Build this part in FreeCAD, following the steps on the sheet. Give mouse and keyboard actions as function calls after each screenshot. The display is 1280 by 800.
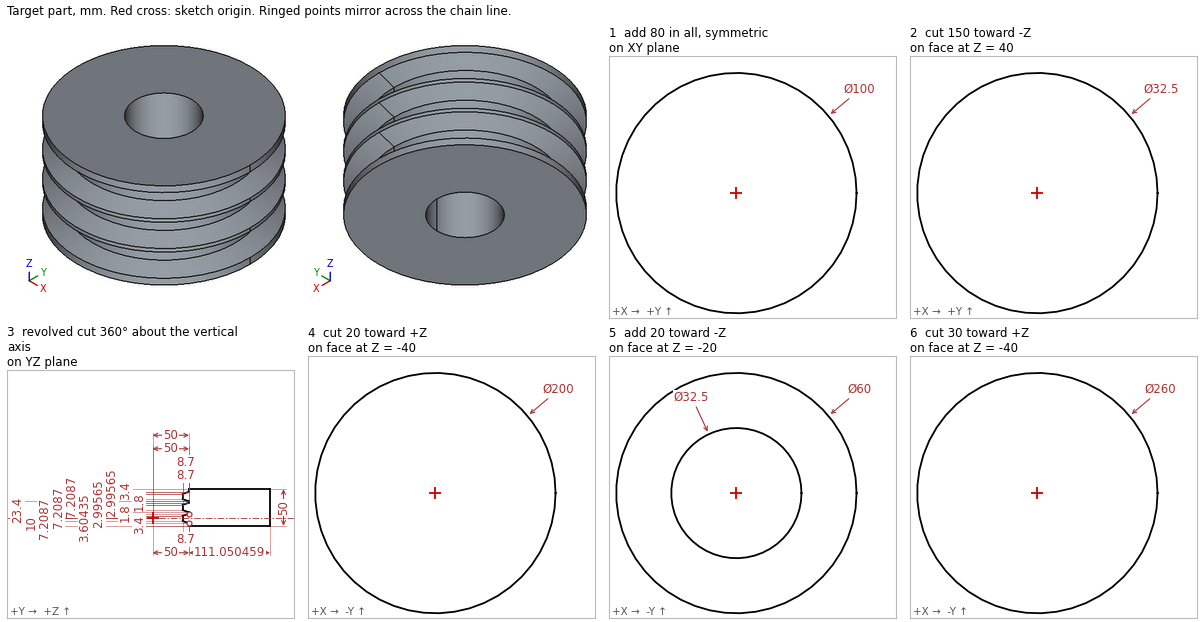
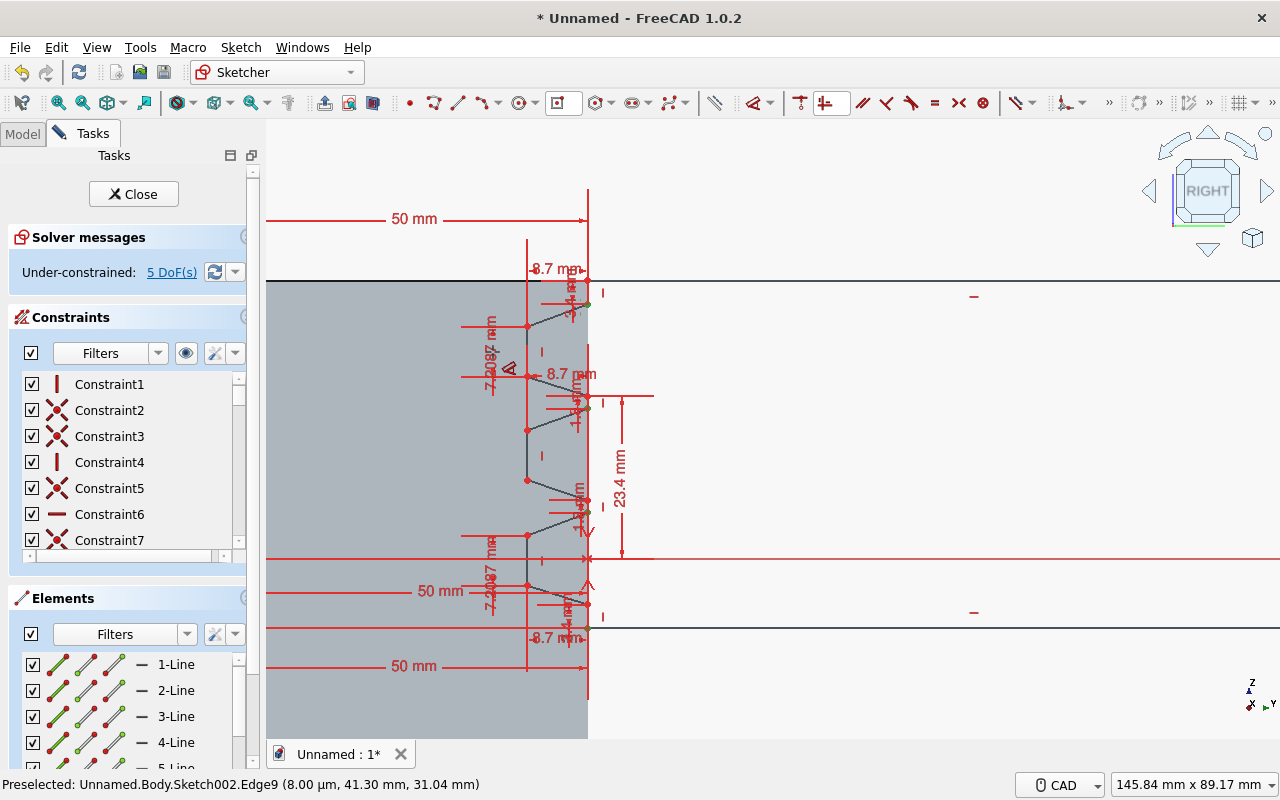
click(527, 445)
click(493, 455)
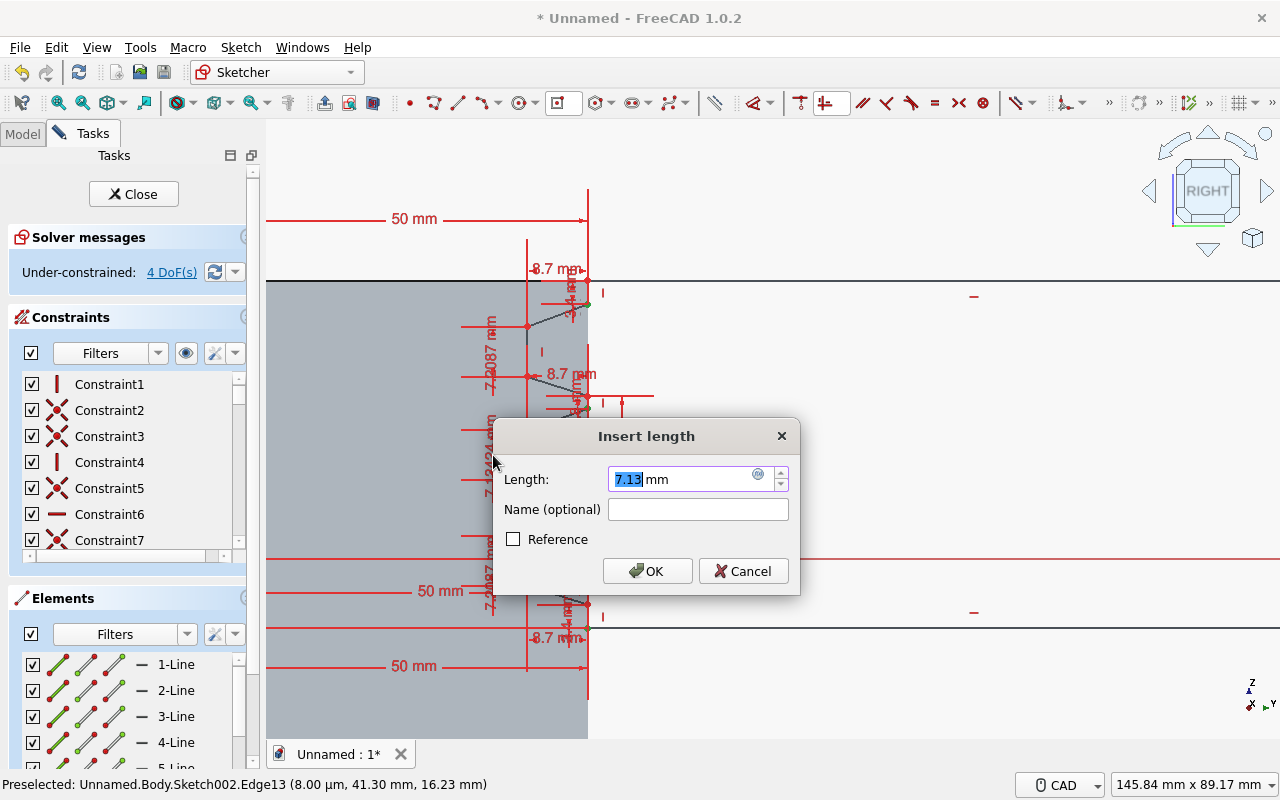
text(7.2087)
key(Return)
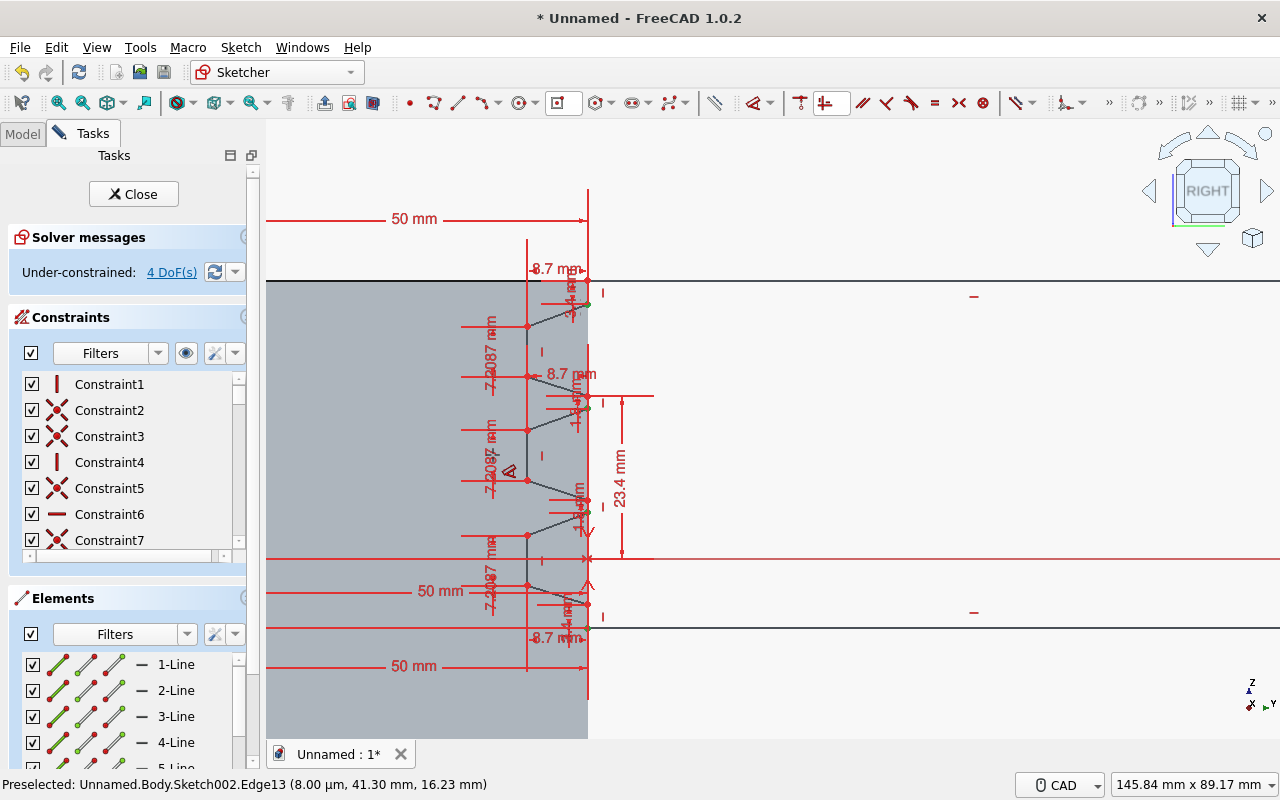
scroll(527, 536, up, 3)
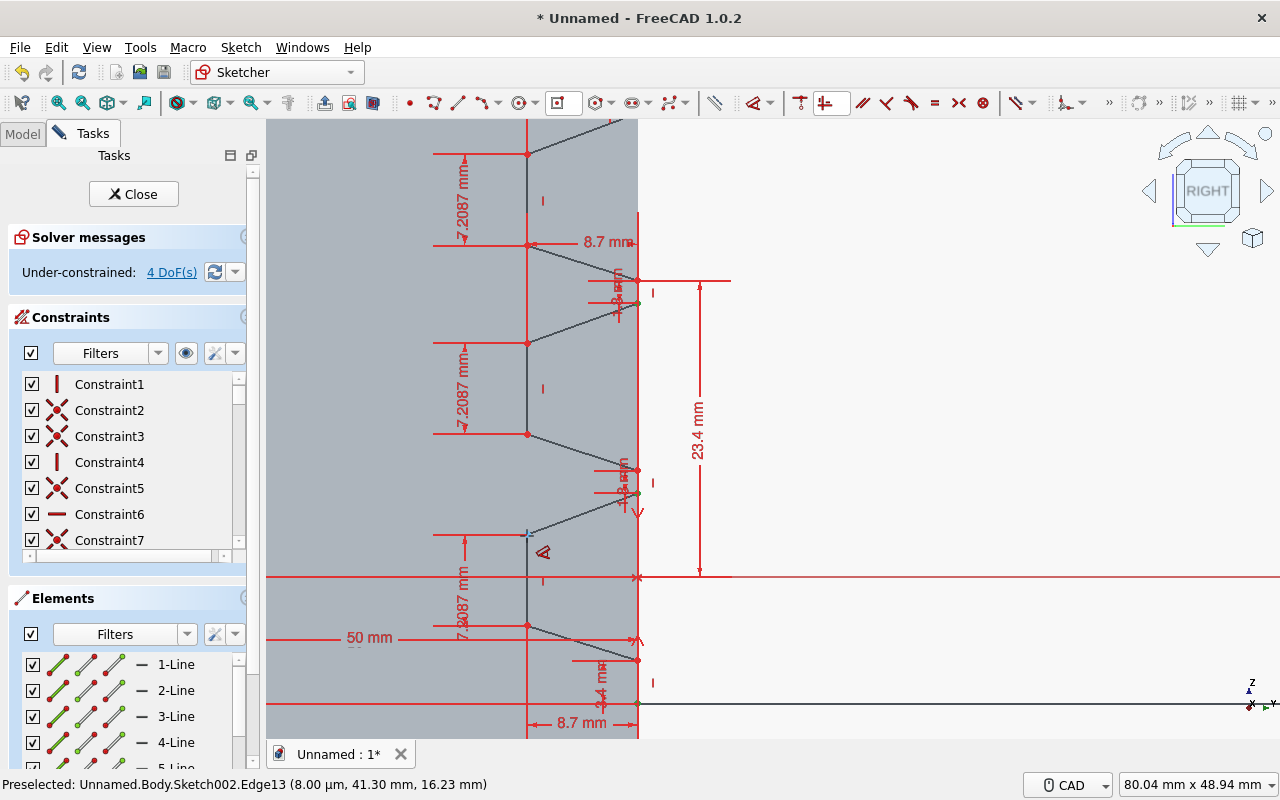
click(528, 535)
click(562, 556)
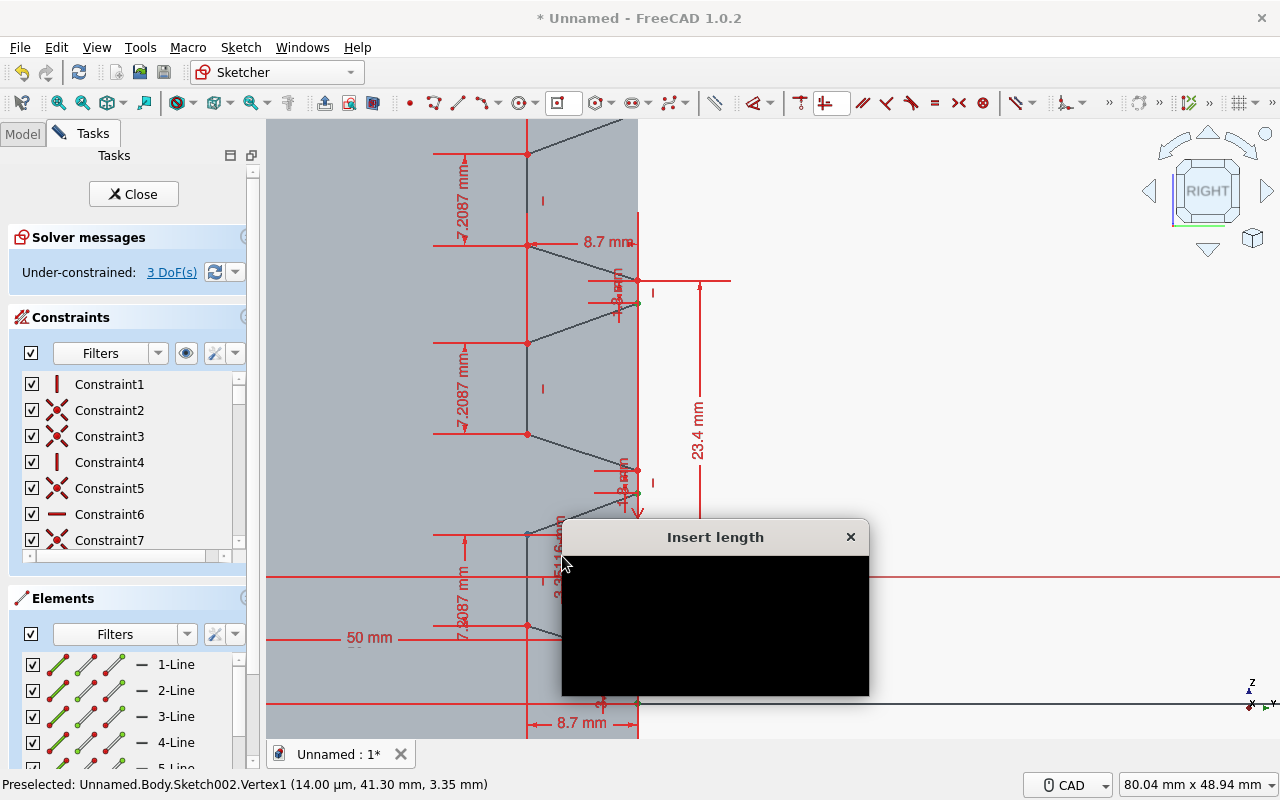
text(3.60435)
key(Return)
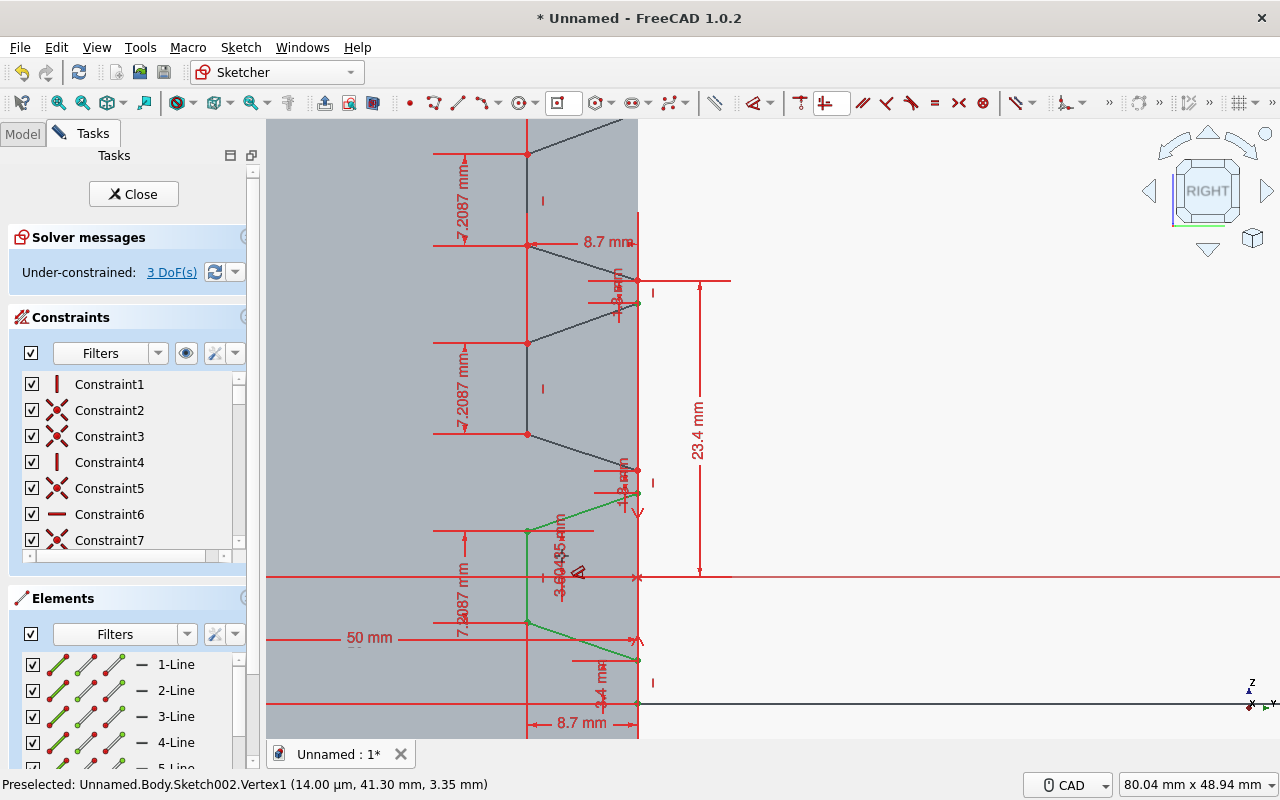
scroll(567, 447, down, 6)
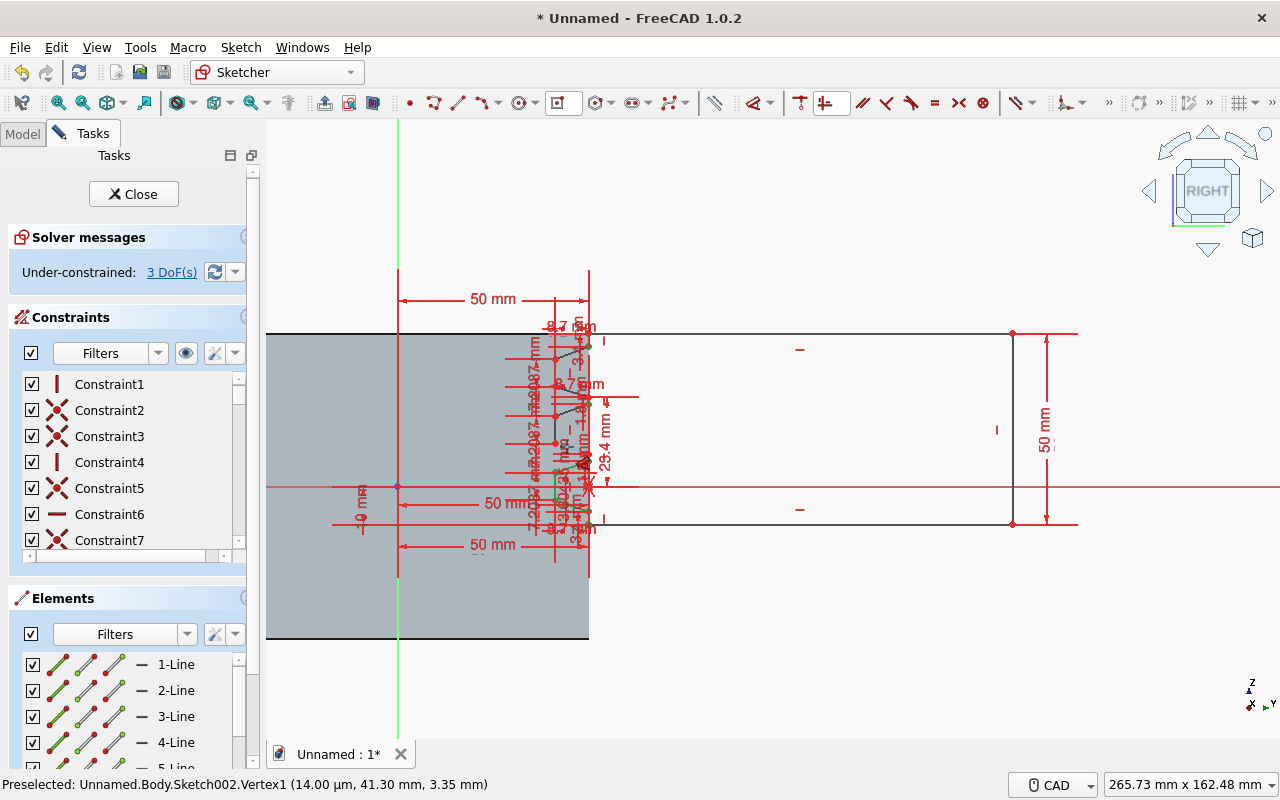
scroll(579, 351, up, 7)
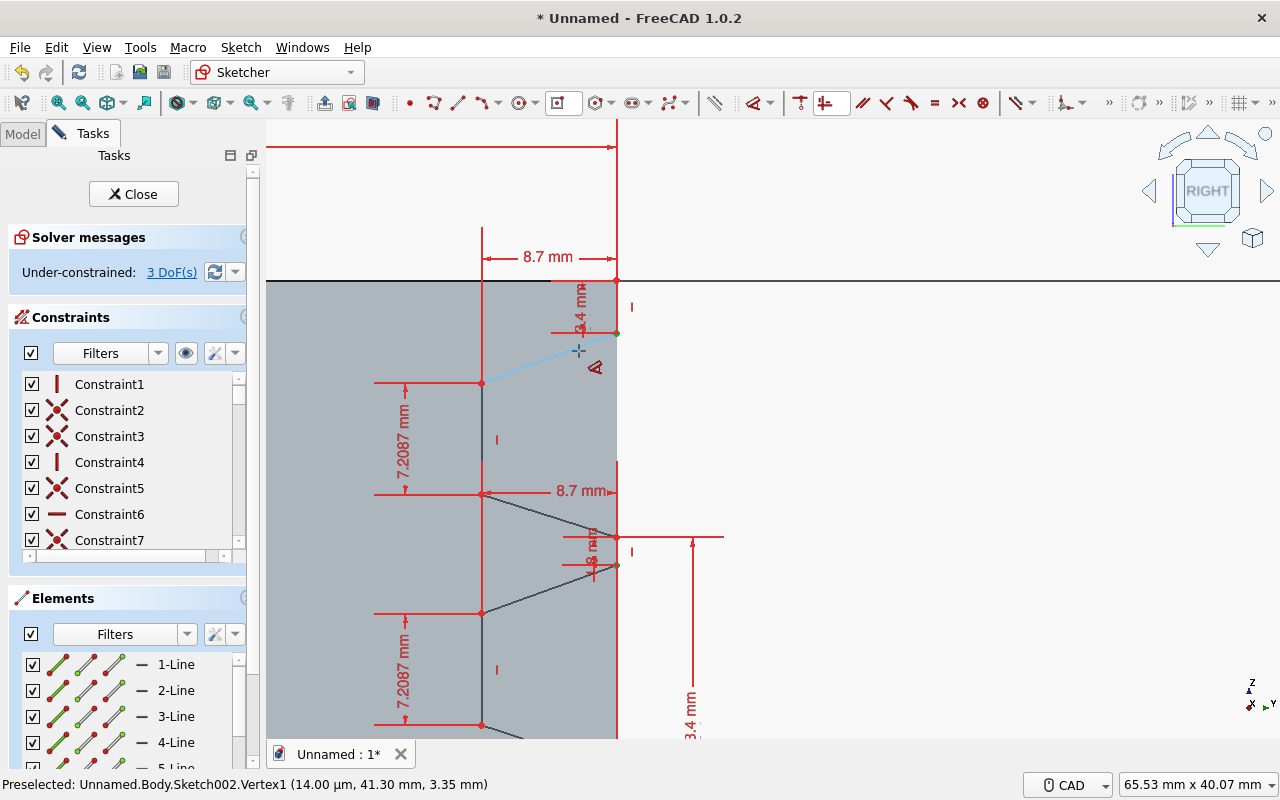
click(576, 348)
click(448, 358)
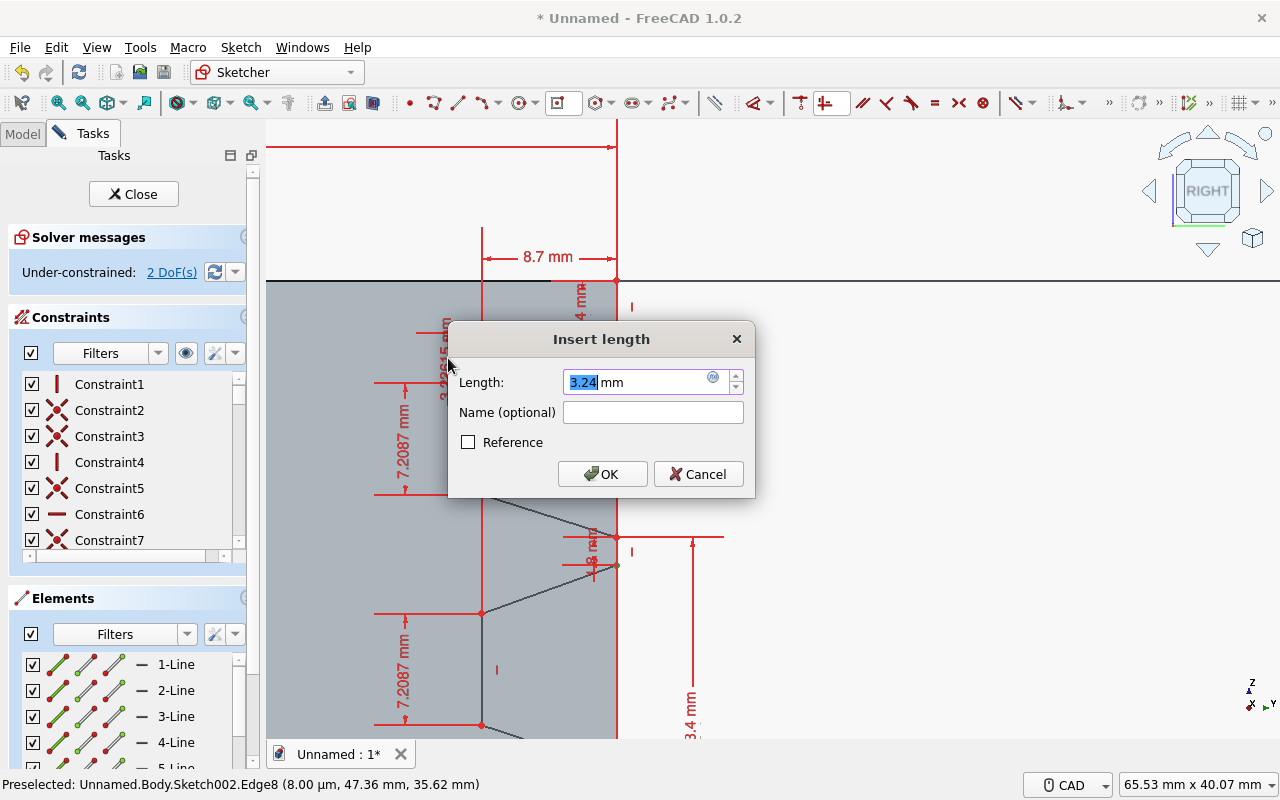
text(2.99565)
key(Return)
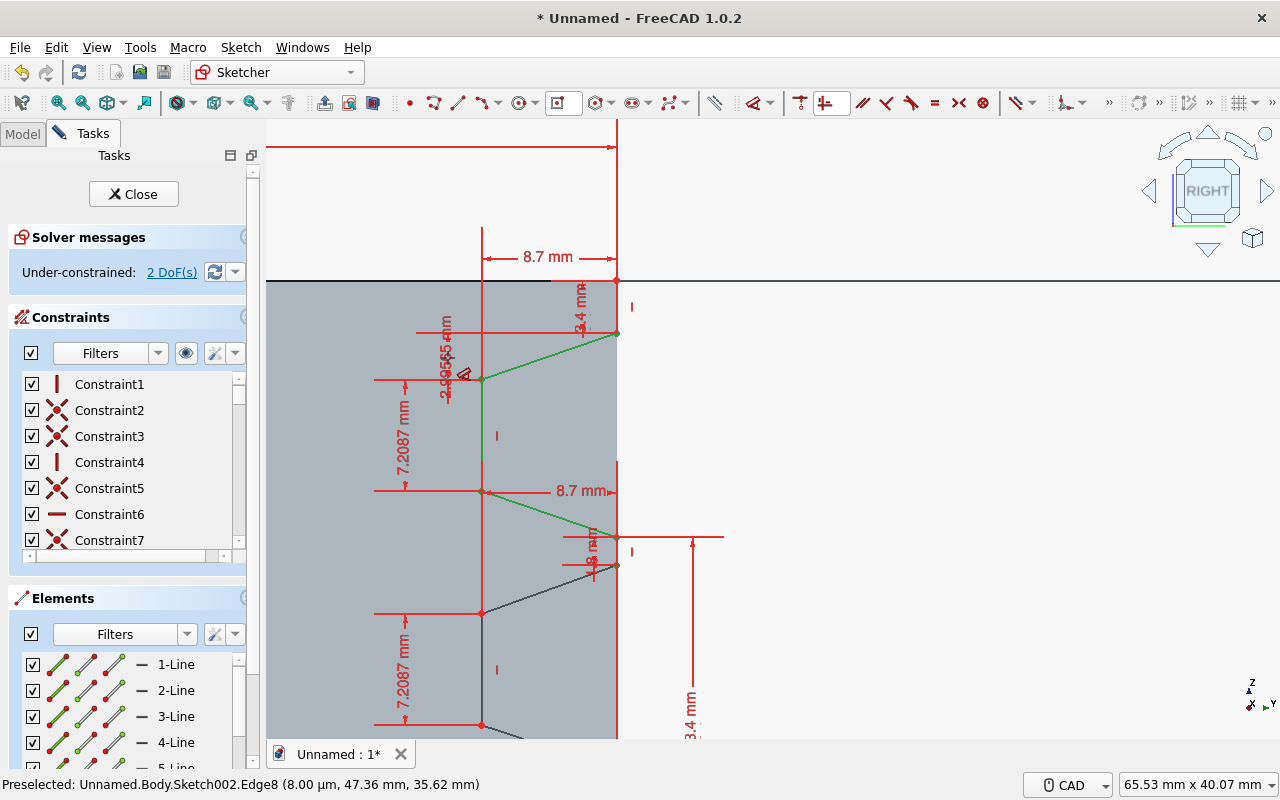
click(576, 580)
click(448, 590)